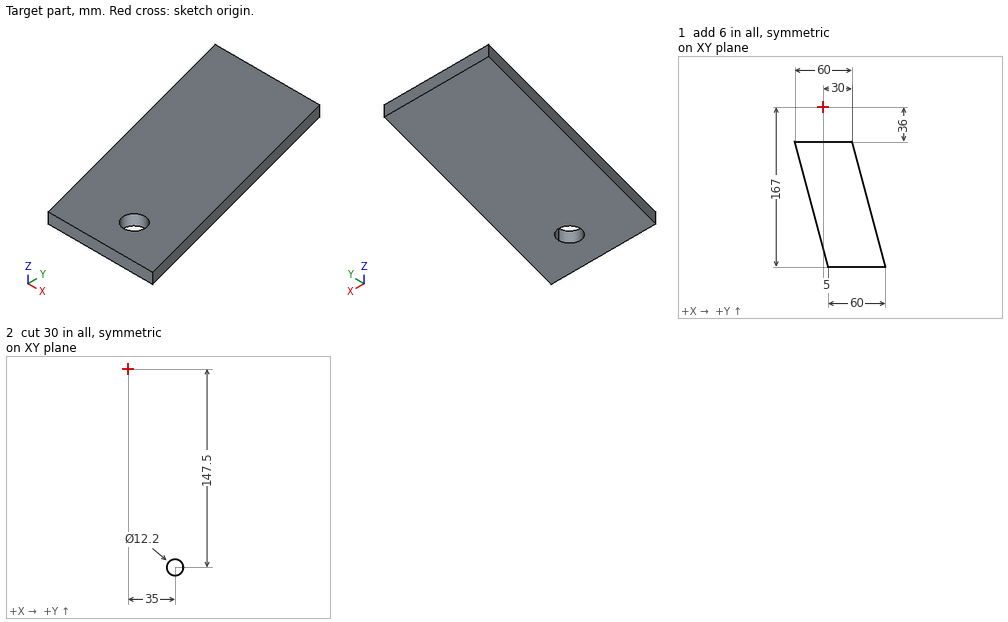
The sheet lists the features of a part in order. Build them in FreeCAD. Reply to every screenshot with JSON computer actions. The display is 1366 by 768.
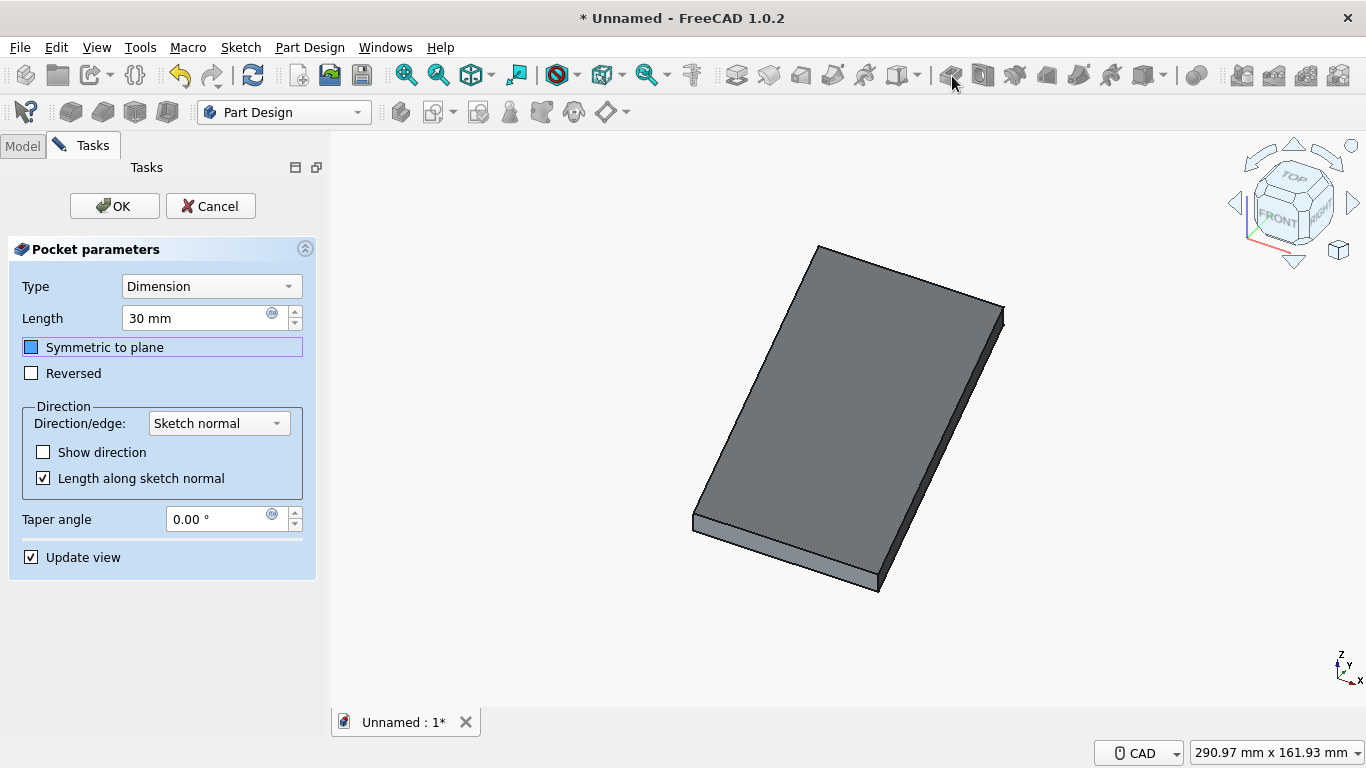
{"action": "left_click", "coordinate": [30, 347]}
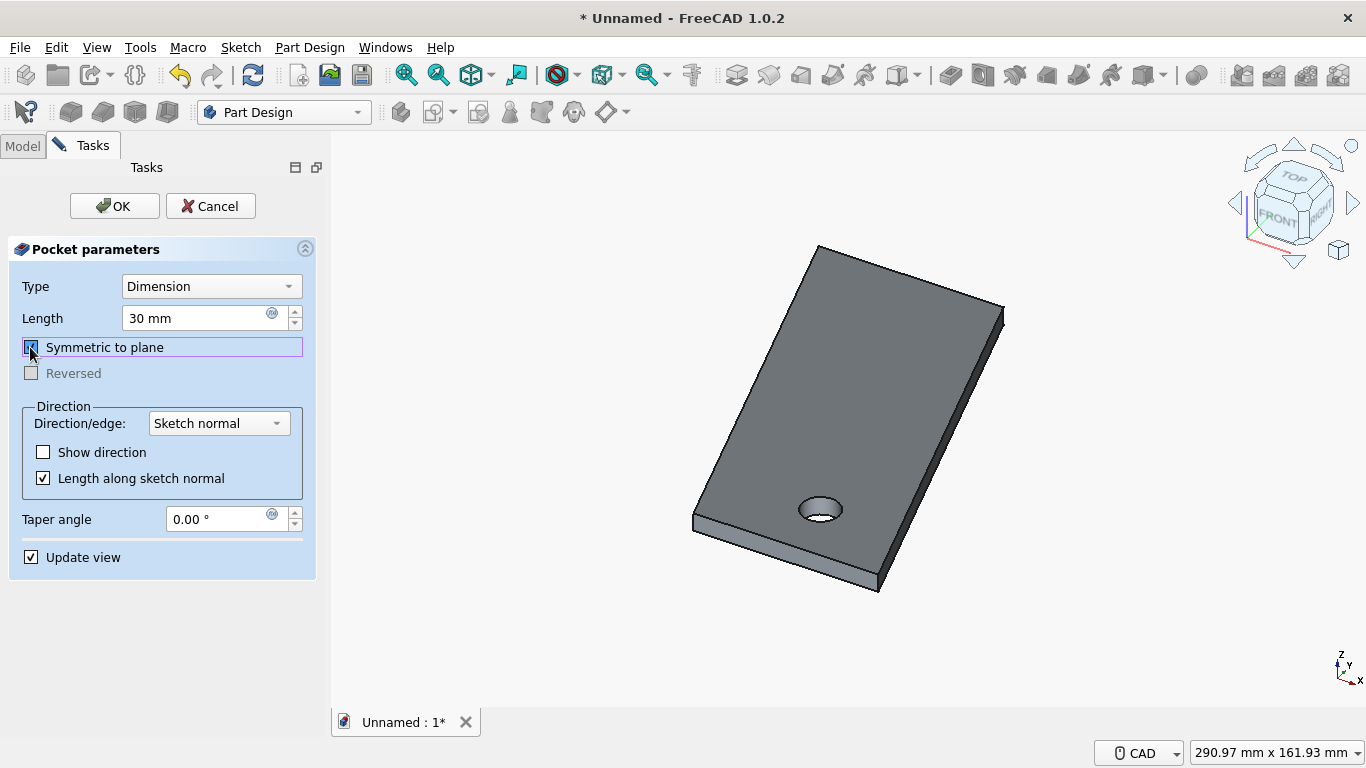
{"action": "left_click", "coordinate": [115, 206]}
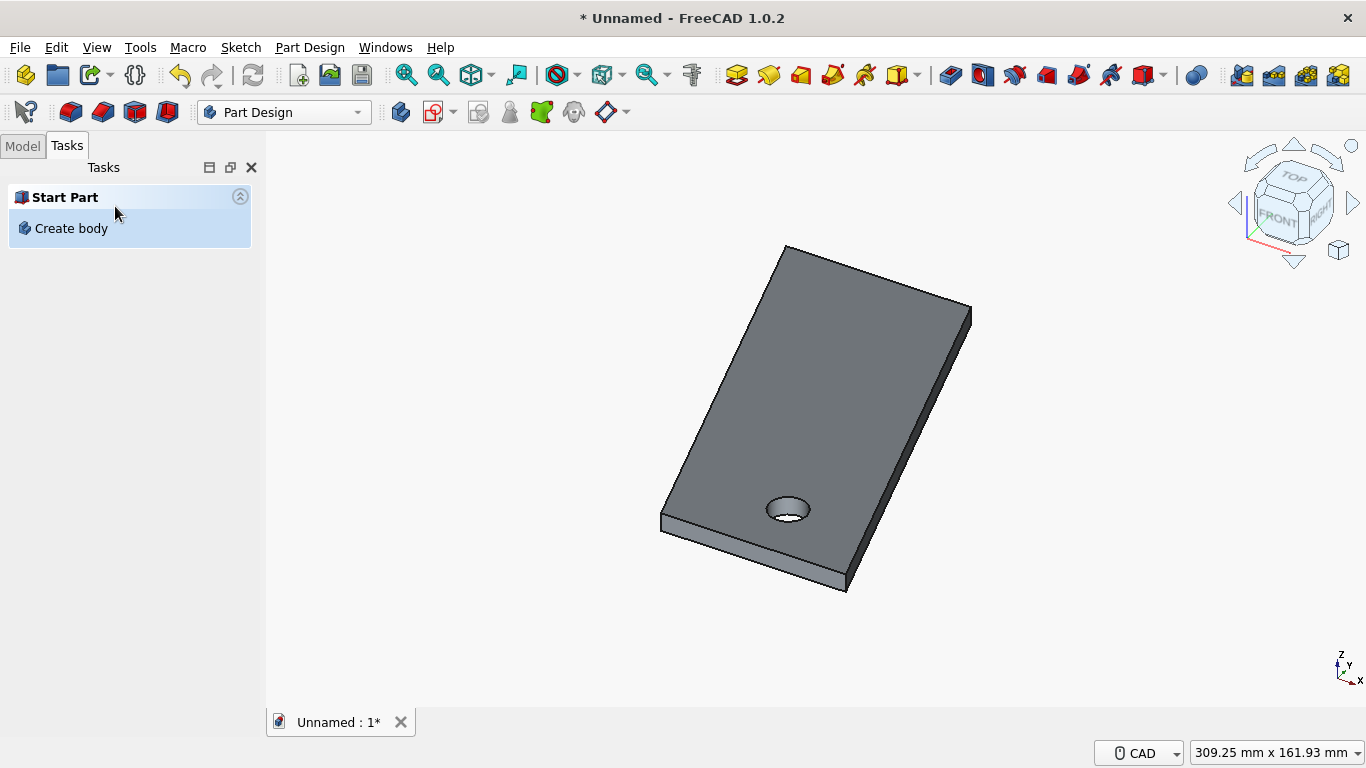
{"action": "key", "text": "0"}